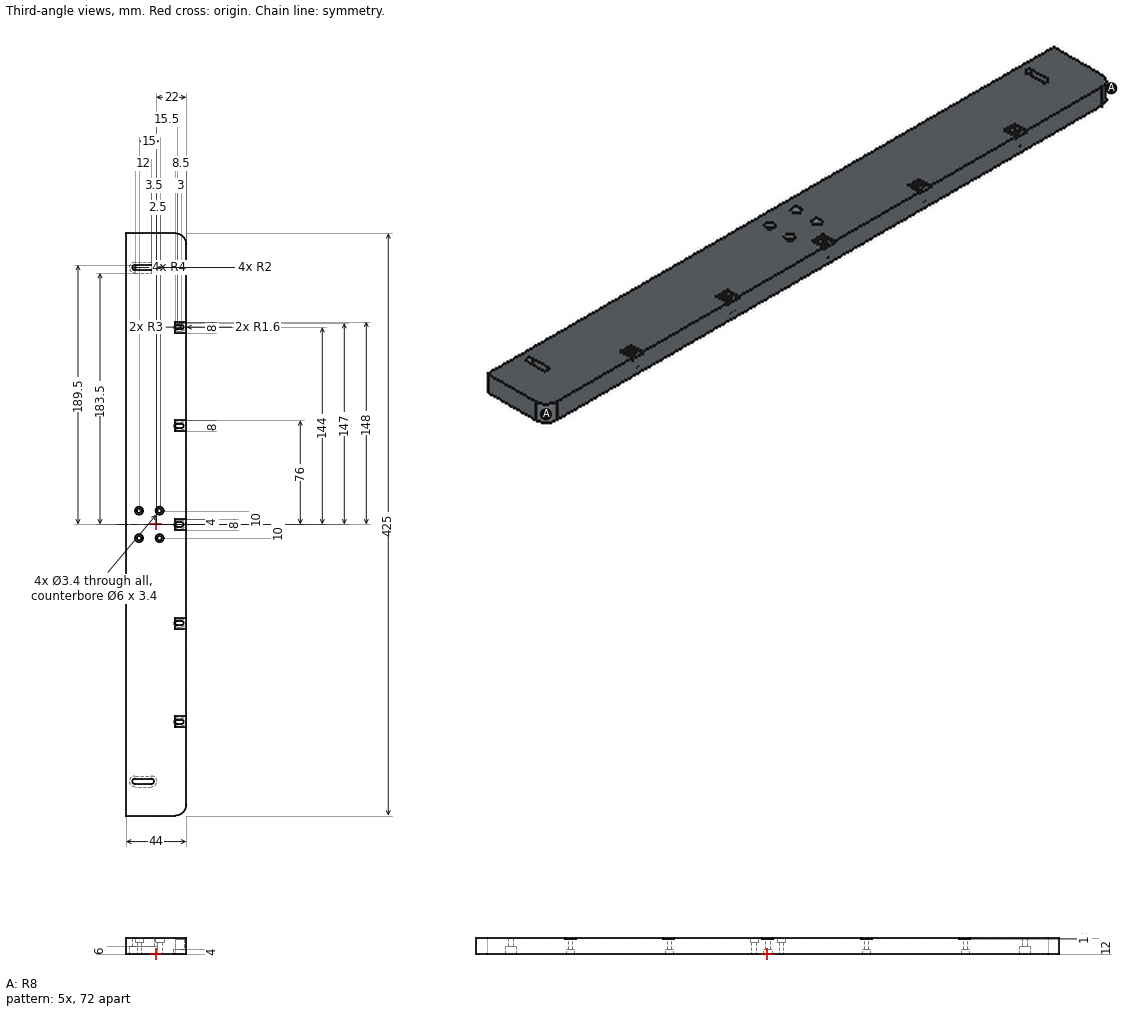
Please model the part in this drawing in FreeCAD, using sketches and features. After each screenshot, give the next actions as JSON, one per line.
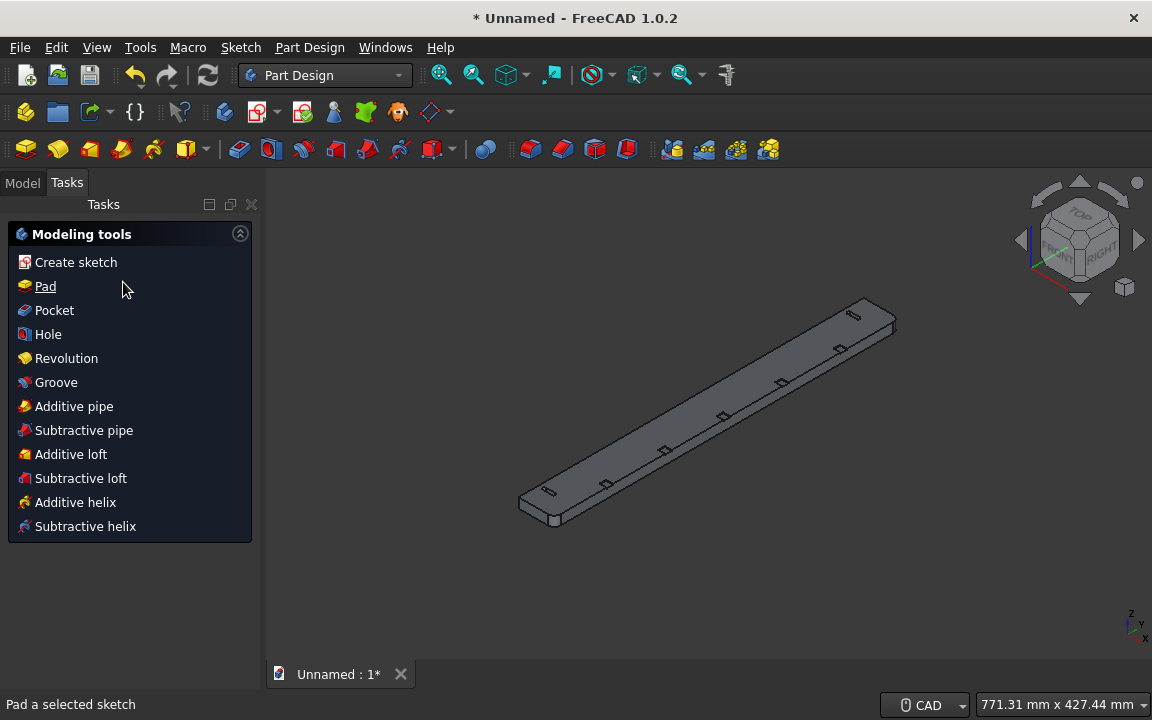
{"action": "left_click", "coordinate": [240, 150]}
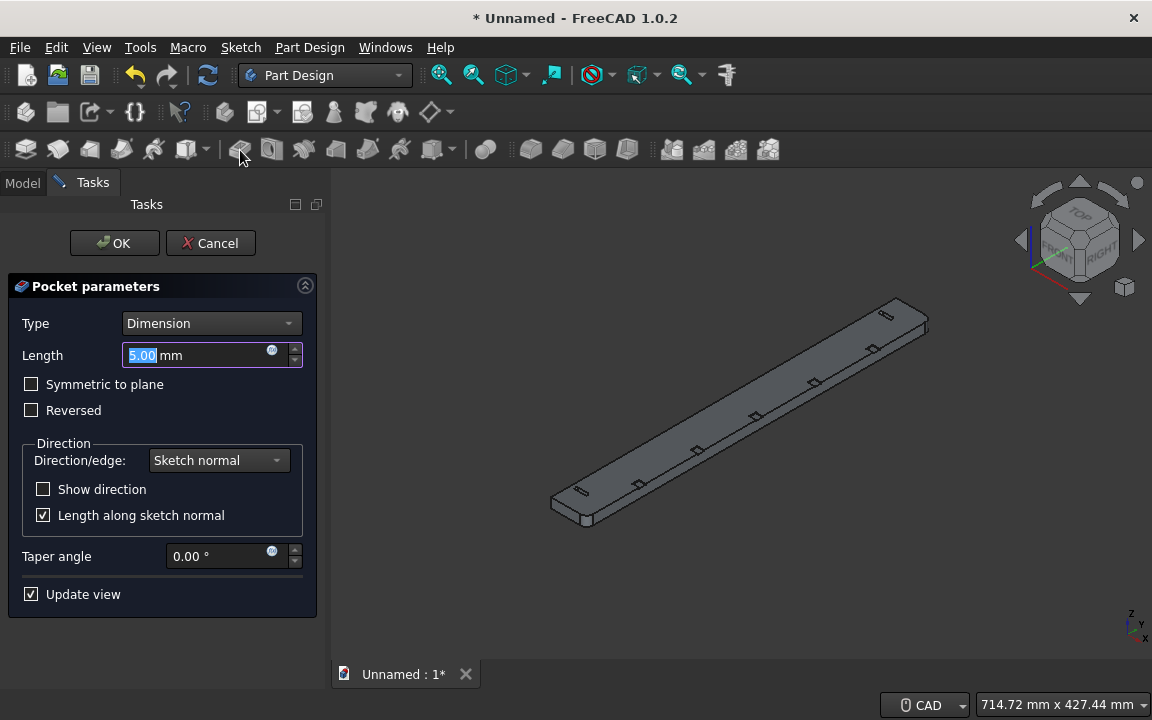
{"action": "type", "text": "4"}
{"action": "key", "text": "Tab"}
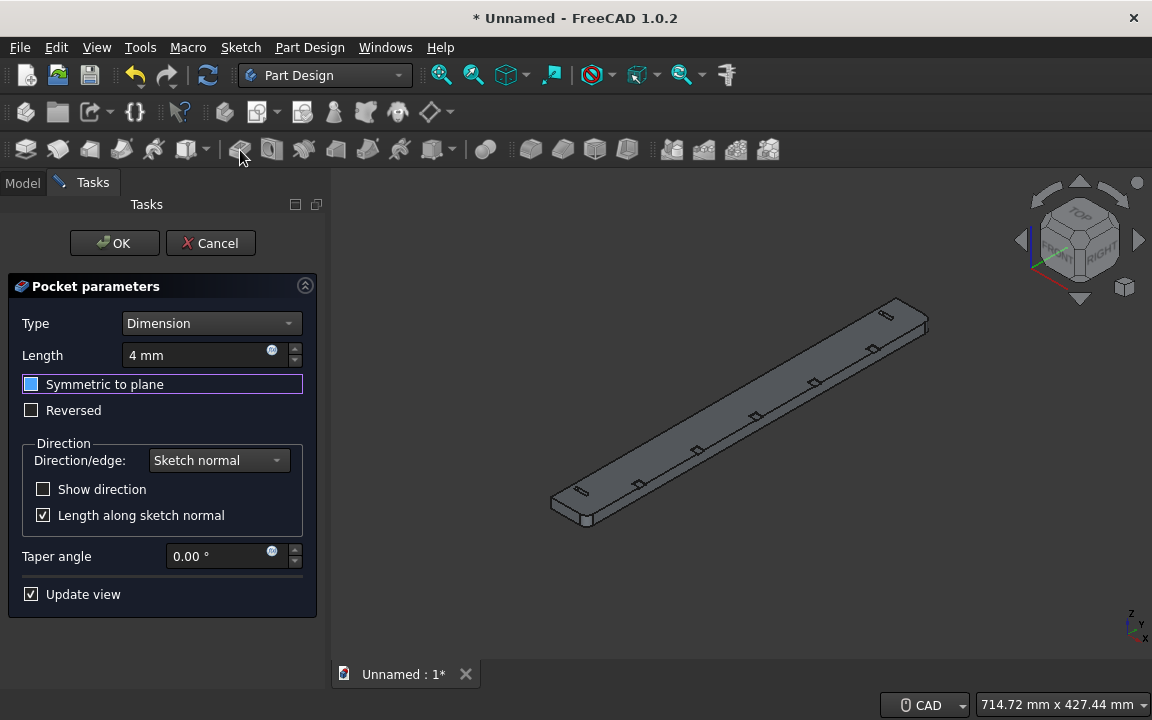
{"action": "left_click", "coordinate": [30, 410]}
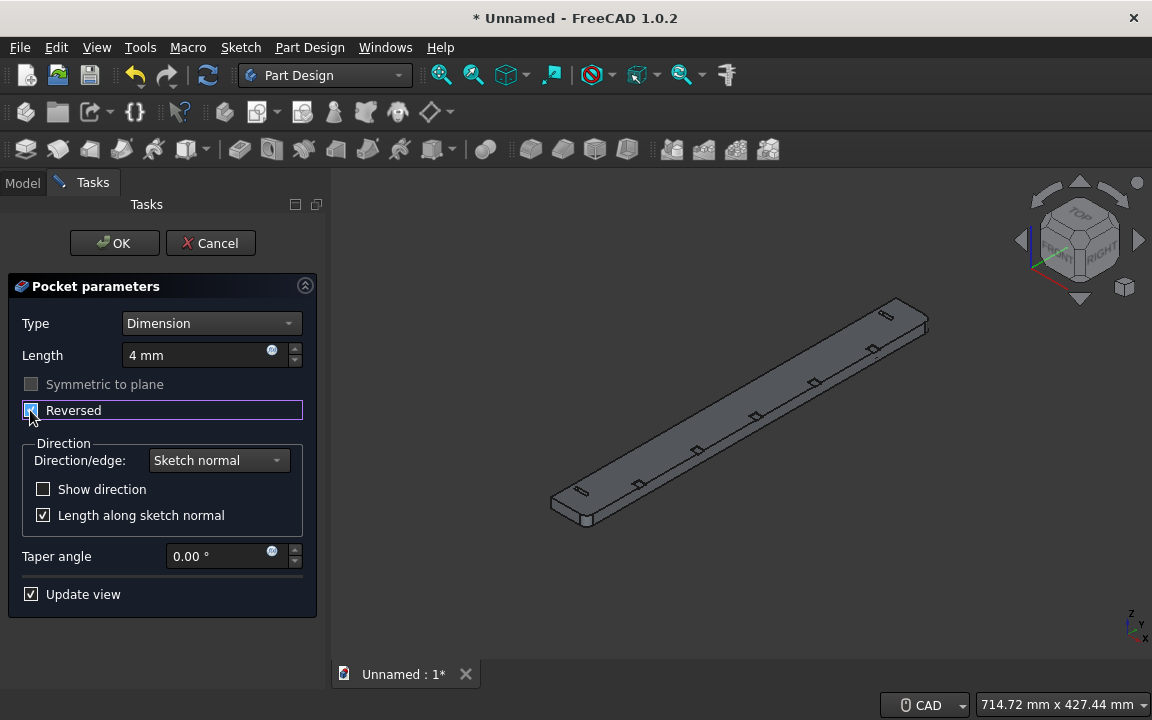
{"action": "left_click", "coordinate": [115, 243]}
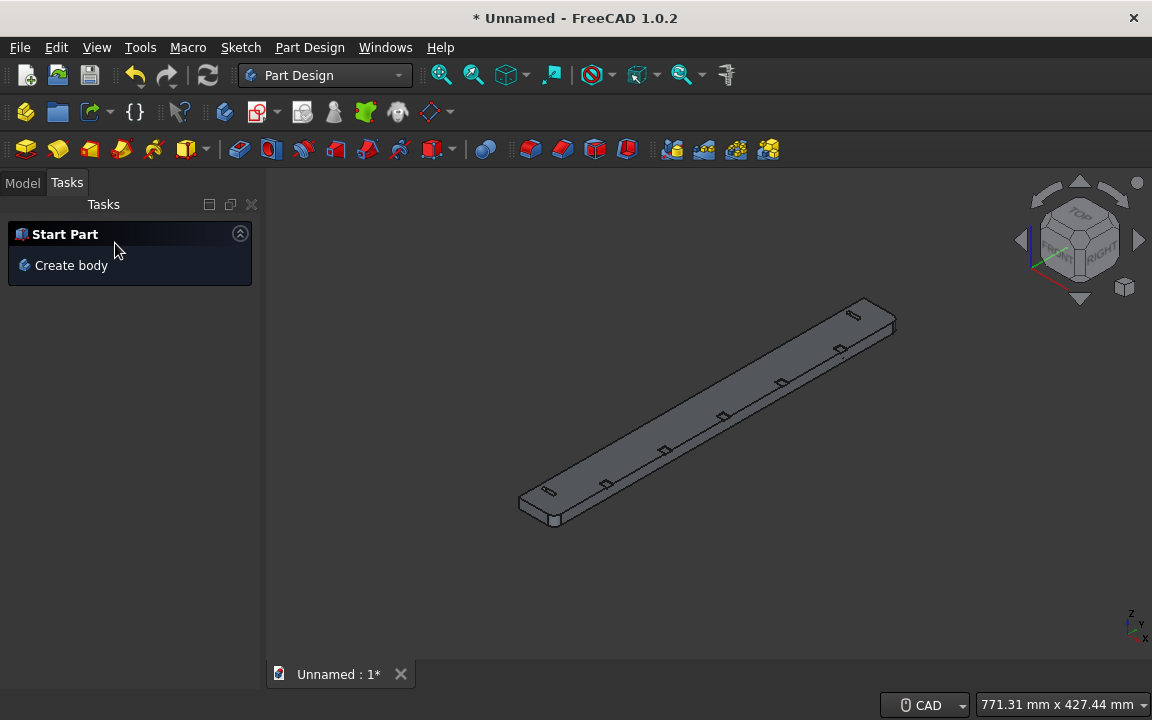
{"action": "key", "text": "5"}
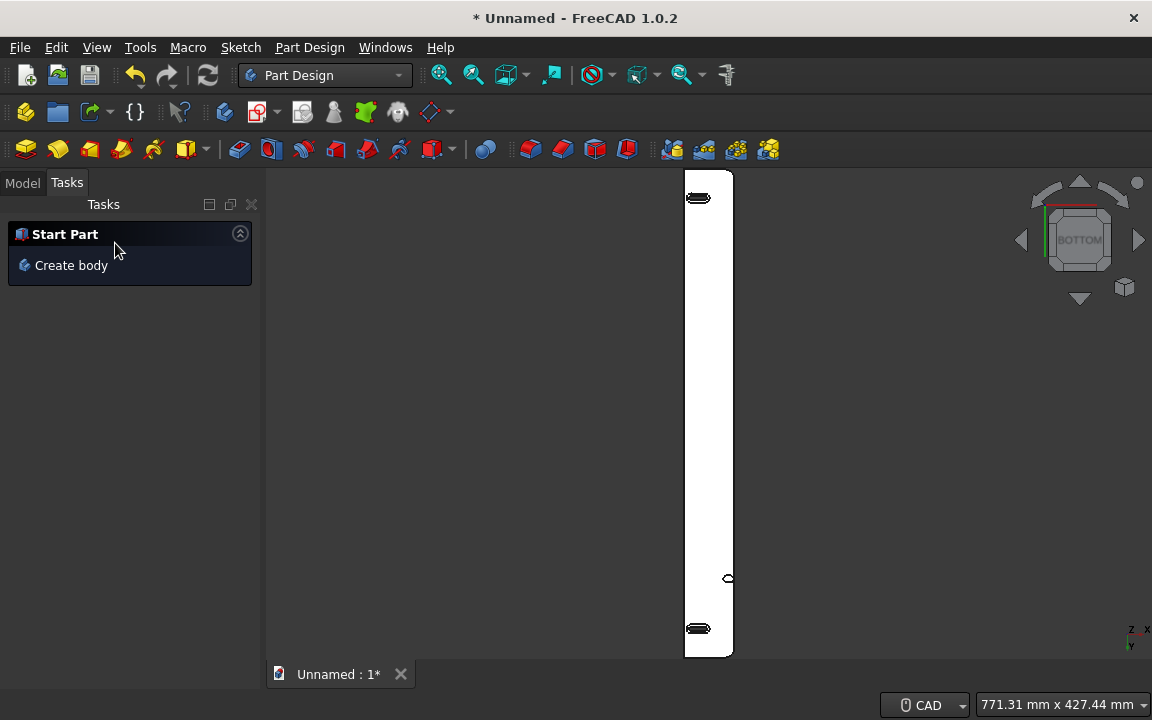
{"action": "scroll", "coordinate": [730, 578], "scroll_direction": "up", "scroll_amount": 7}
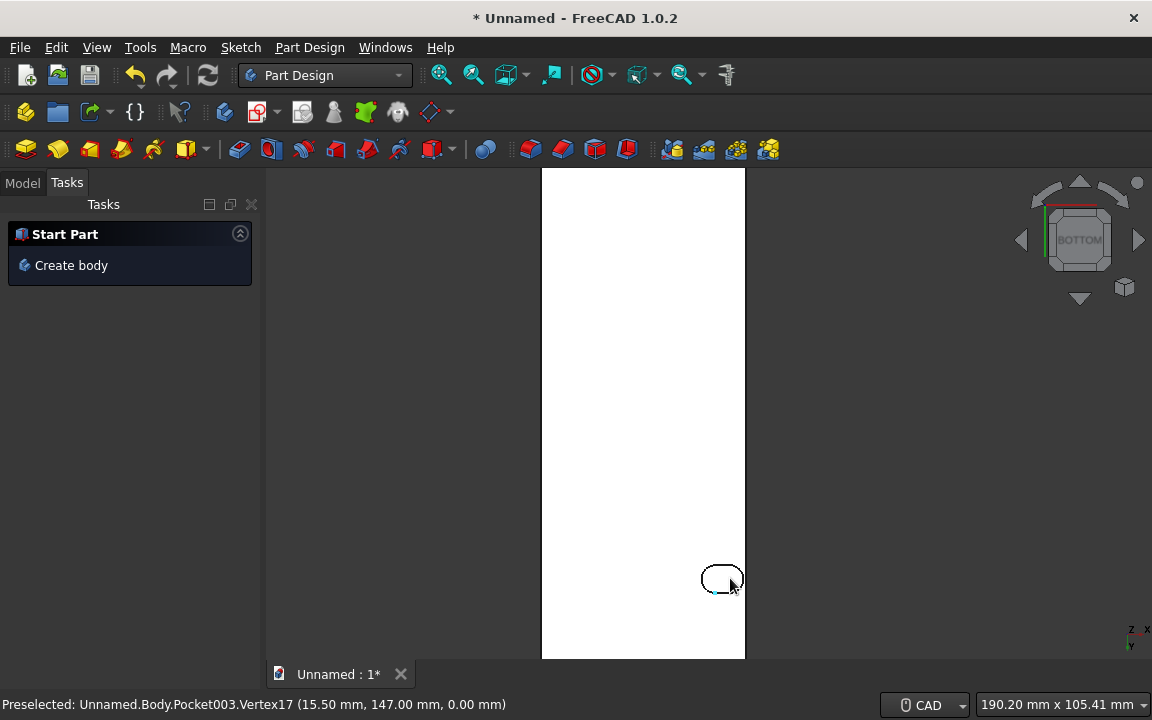
{"action": "left_click", "coordinate": [728, 578]}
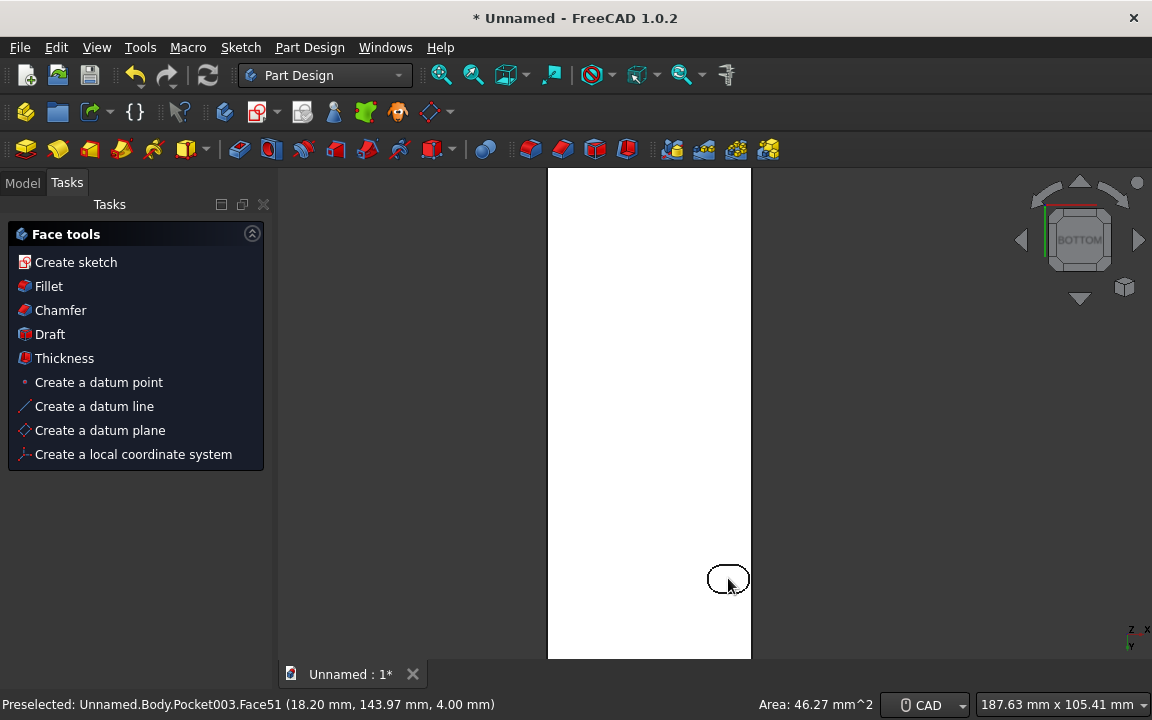
{"action": "left_click", "coordinate": [258, 112]}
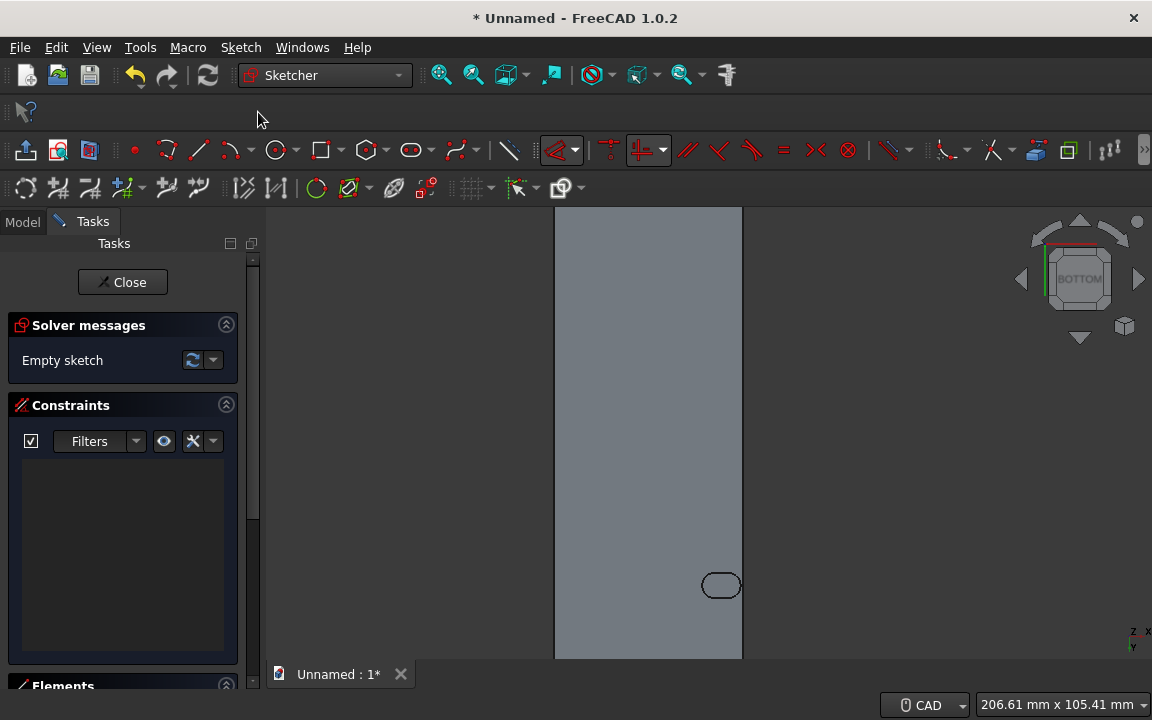
{"action": "key", "text": "q s"}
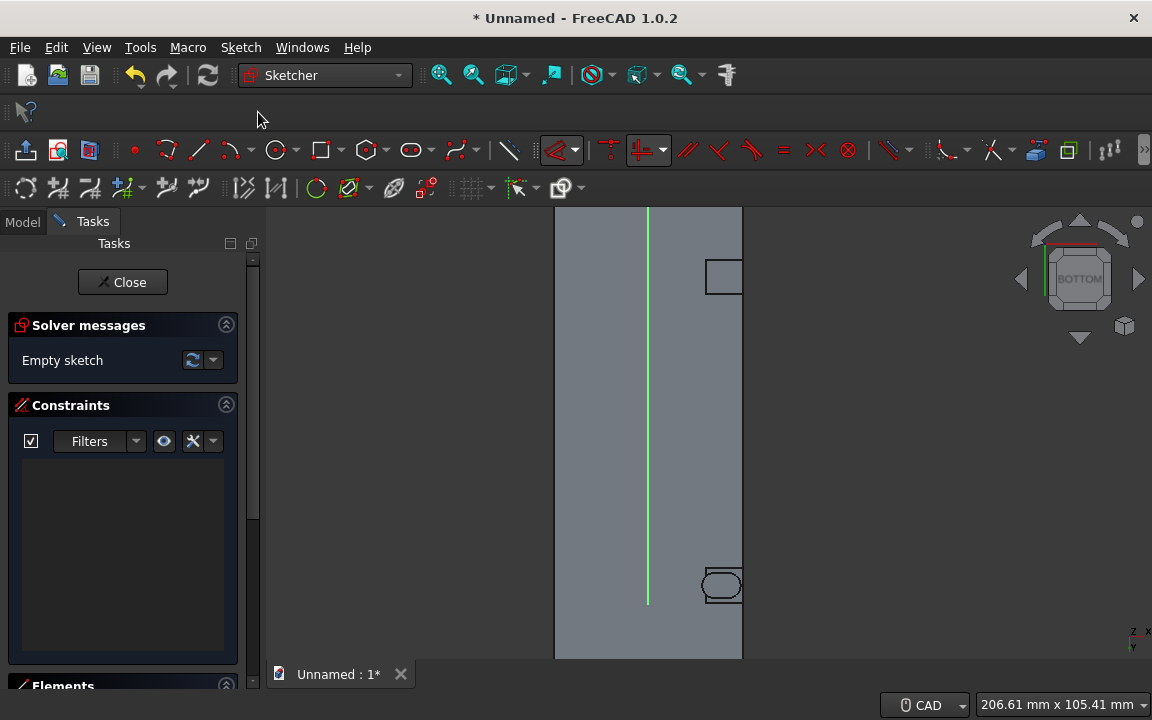
{"action": "scroll", "coordinate": [726, 593], "scroll_direction": "up", "scroll_amount": 15}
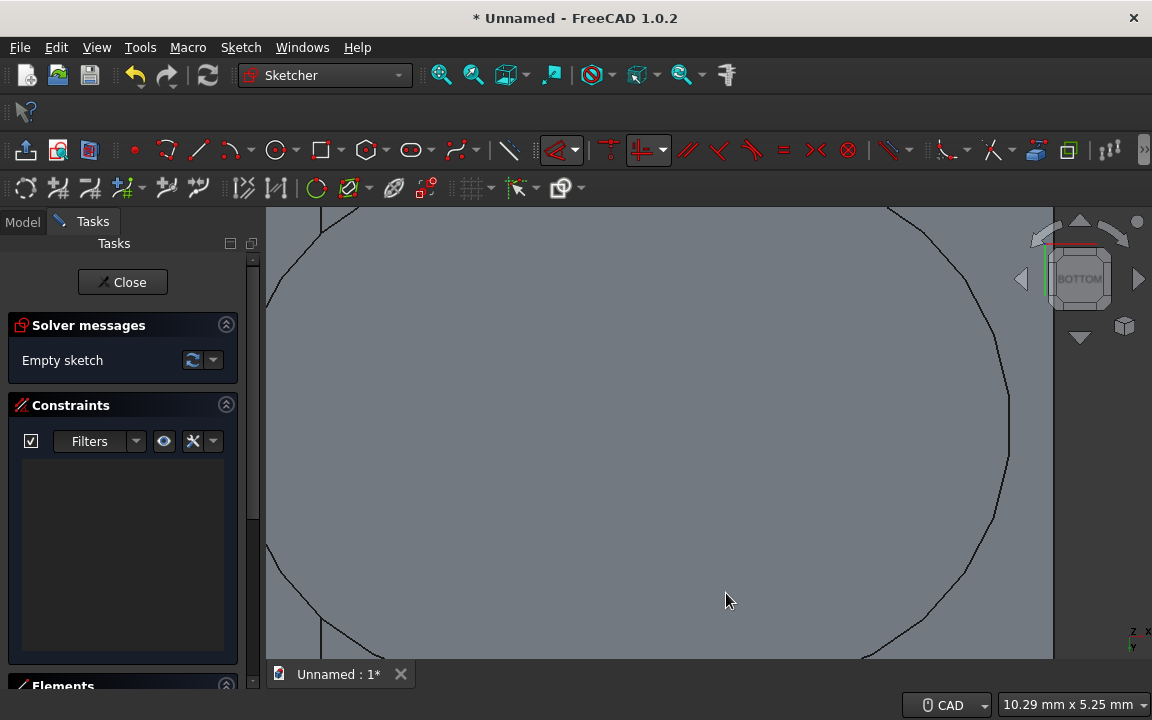
{"action": "key", "text": "g s"}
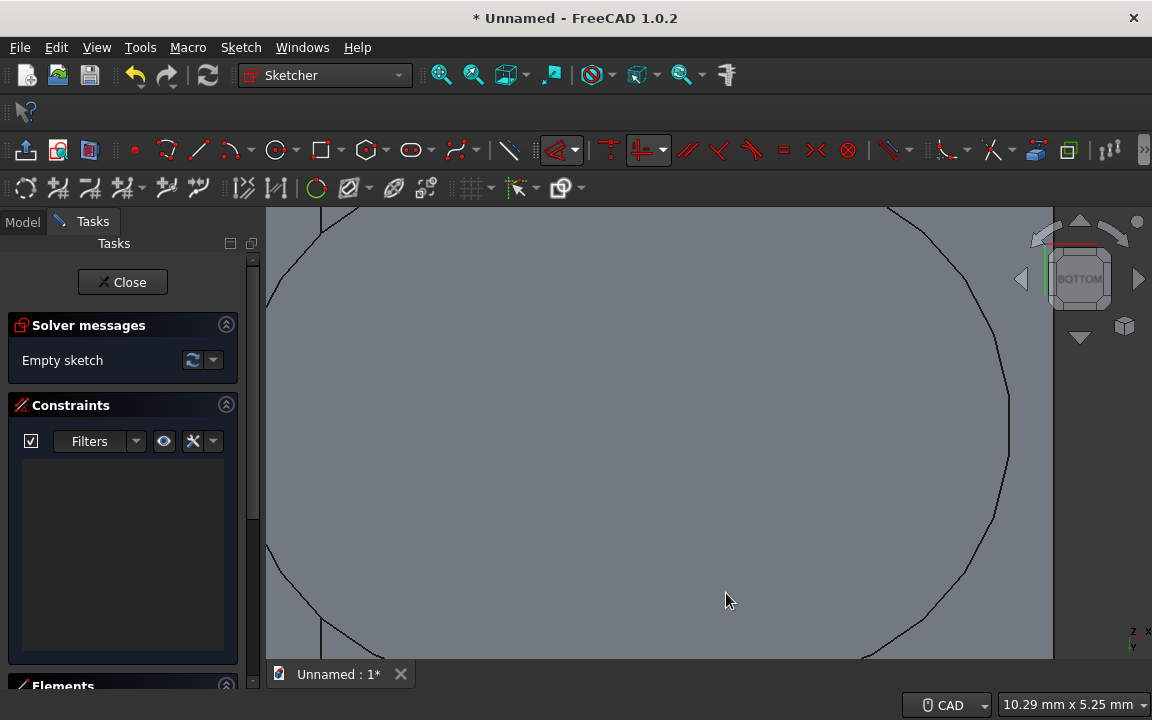
{"action": "left_click", "coordinate": [494, 426]}